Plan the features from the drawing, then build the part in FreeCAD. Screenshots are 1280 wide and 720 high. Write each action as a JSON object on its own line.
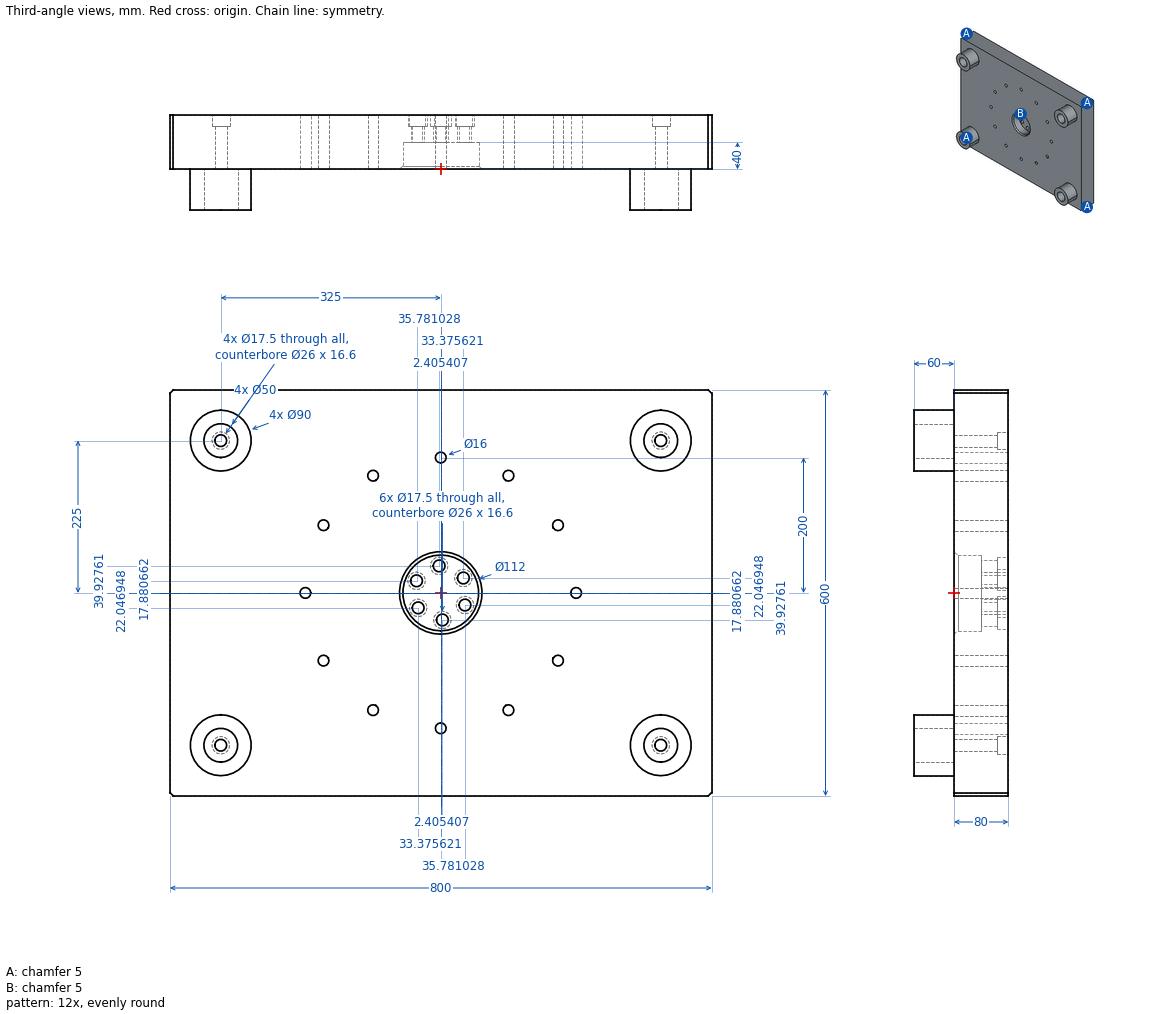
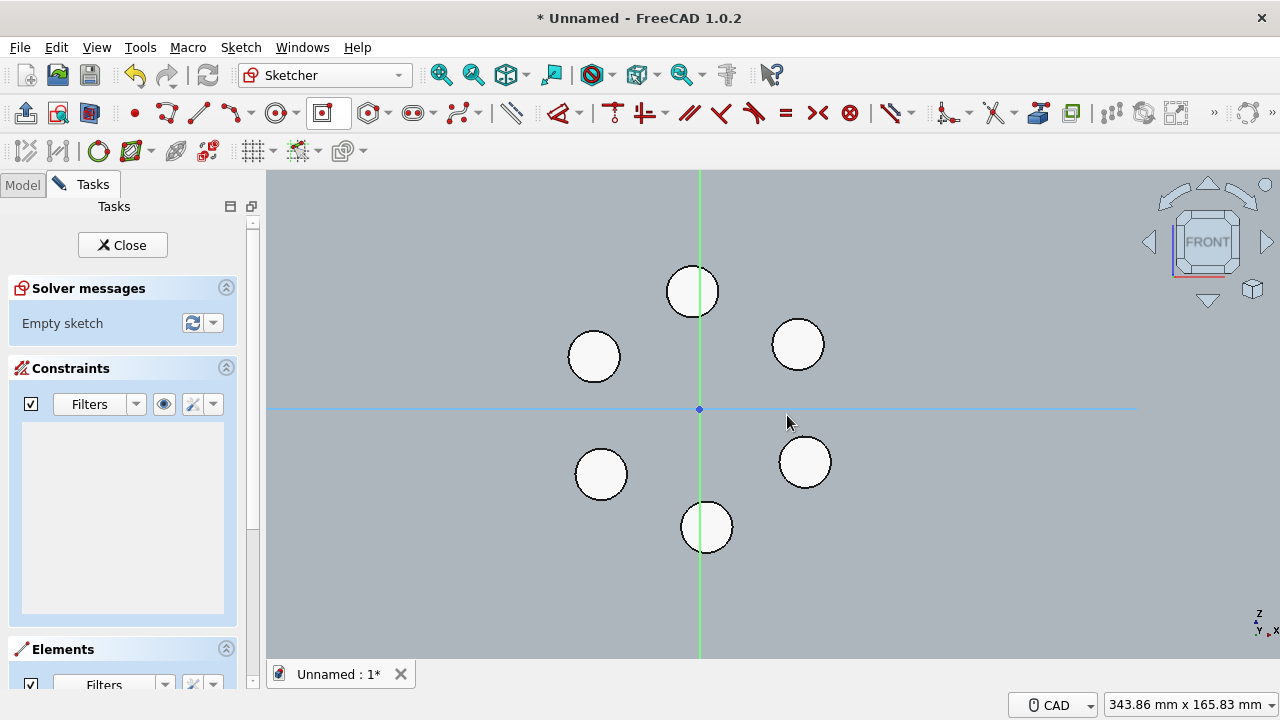
{"action": "left_click", "coordinate": [276, 114]}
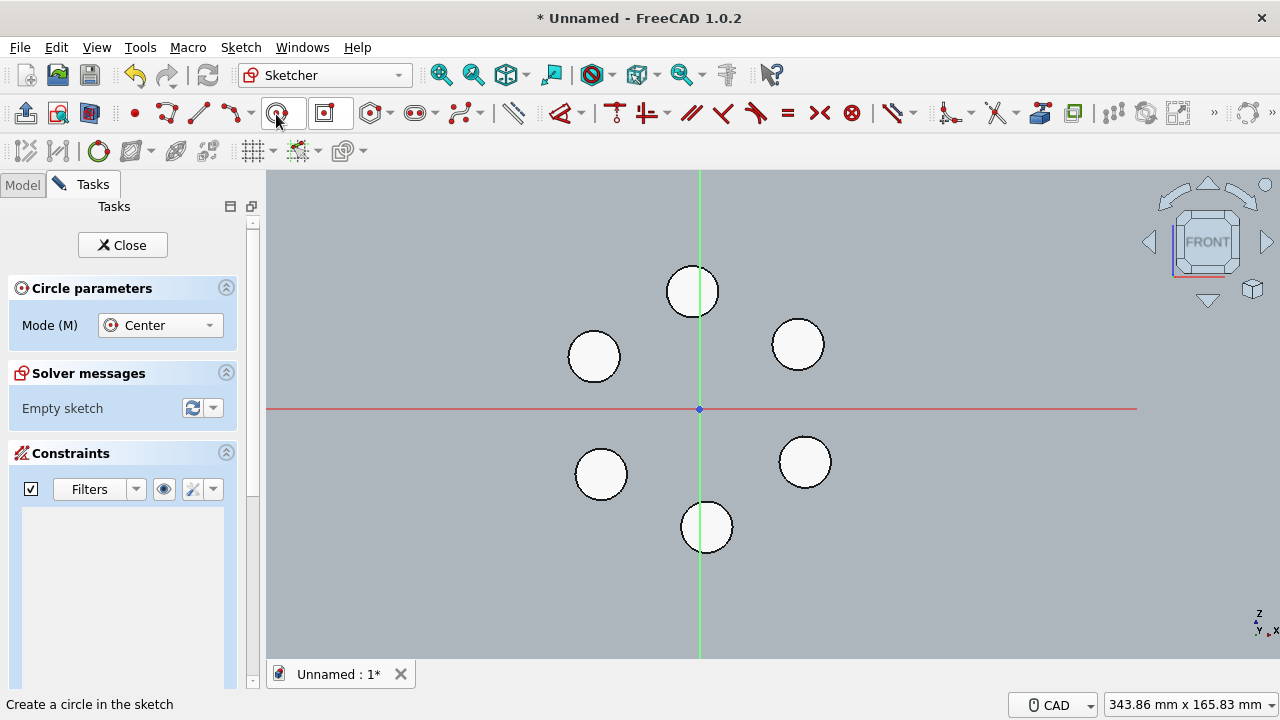
{"action": "left_click", "coordinate": [700, 409]}
{"action": "mouse_move", "coordinate": [816, 293]}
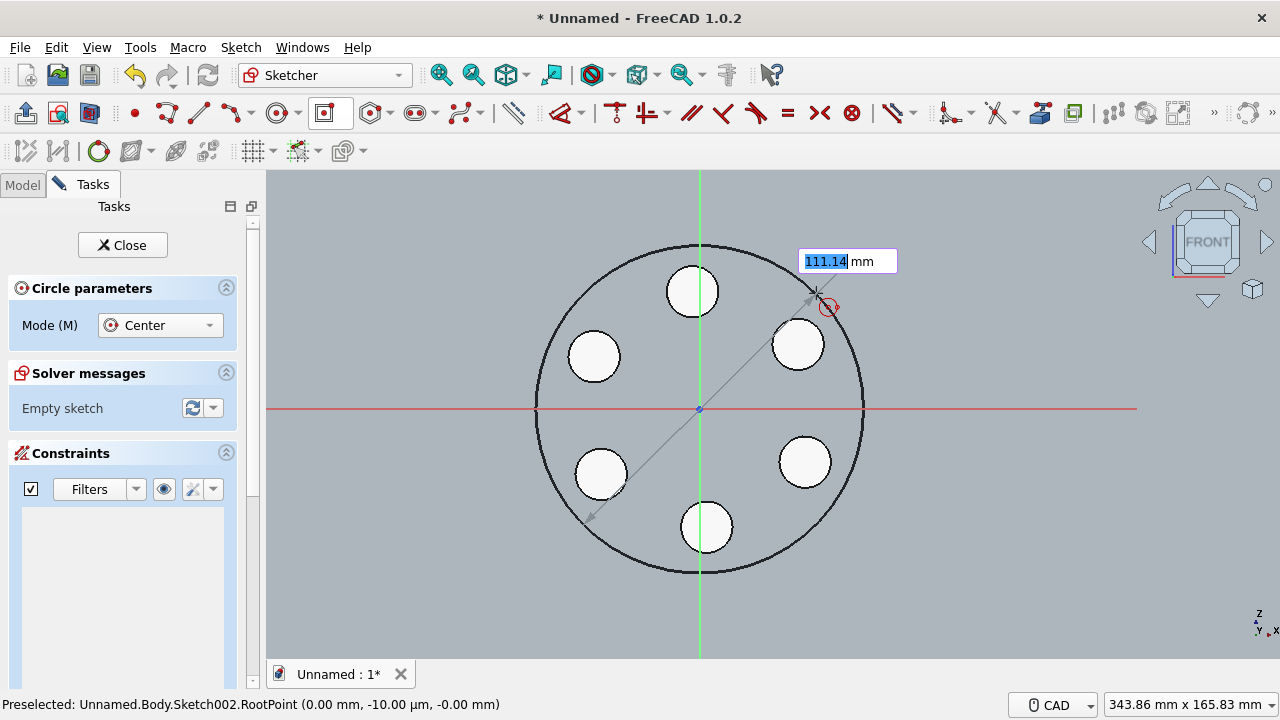
{"action": "type", "text": "112"}
{"action": "key", "text": "Return"}
{"action": "key", "text": "Escape"}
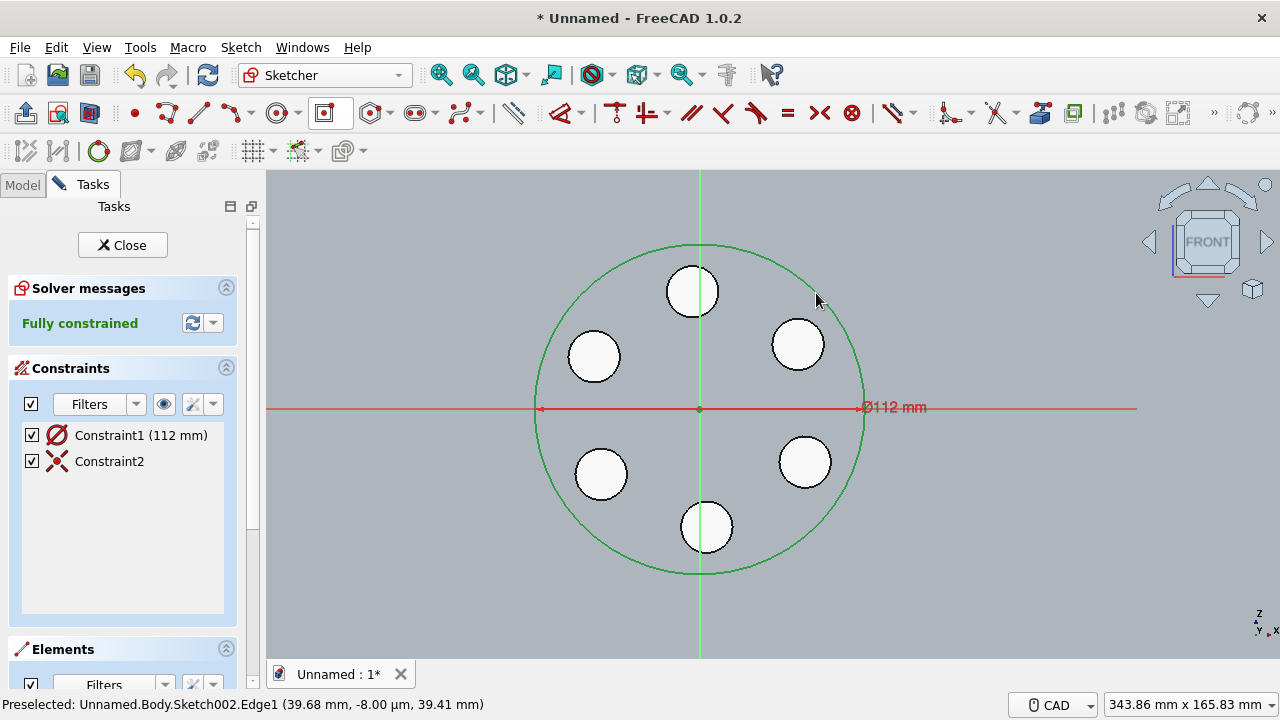
{"action": "left_click", "coordinate": [123, 245]}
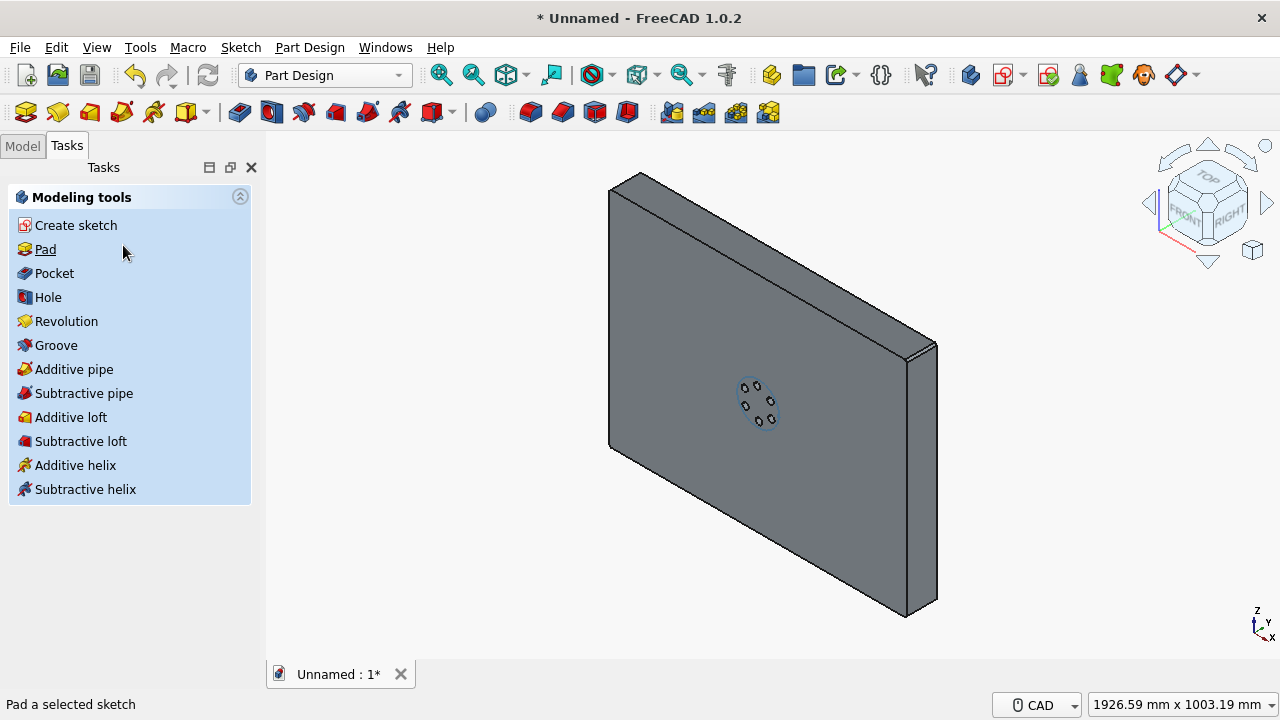
{"action": "left_click", "coordinate": [240, 112]}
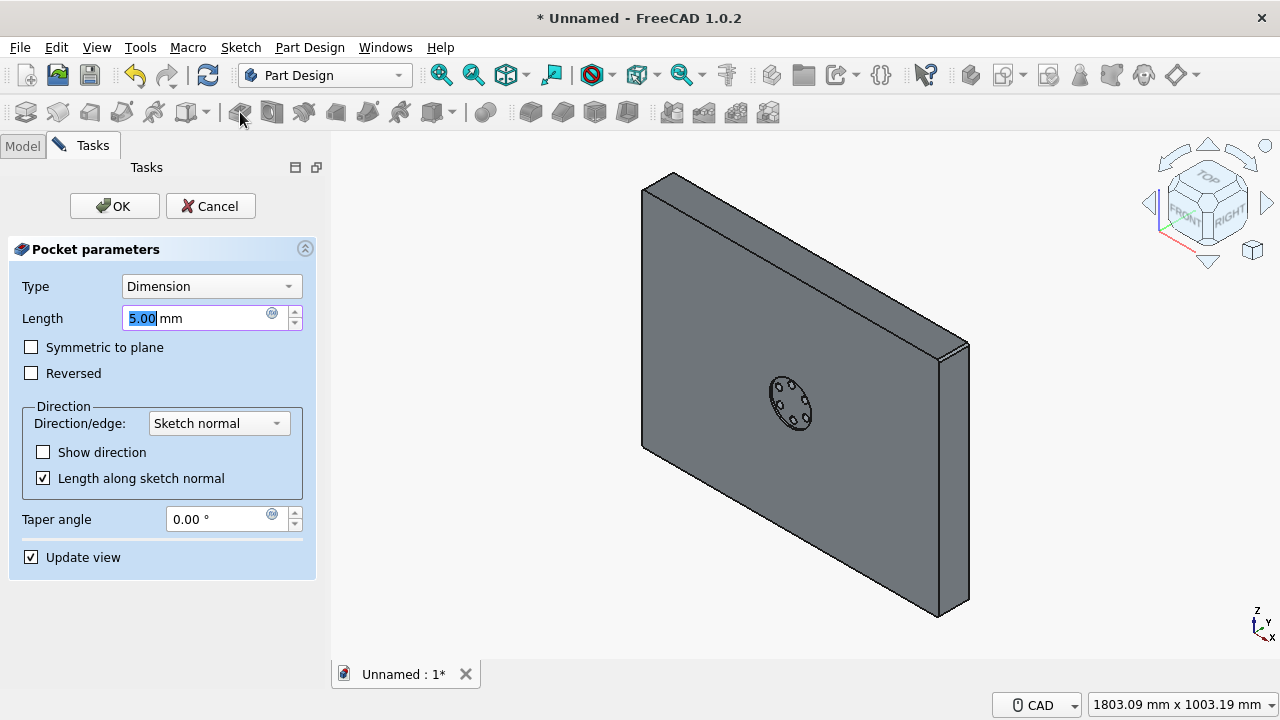
{"action": "type", "text": "40"}
{"action": "key", "text": "Tab"}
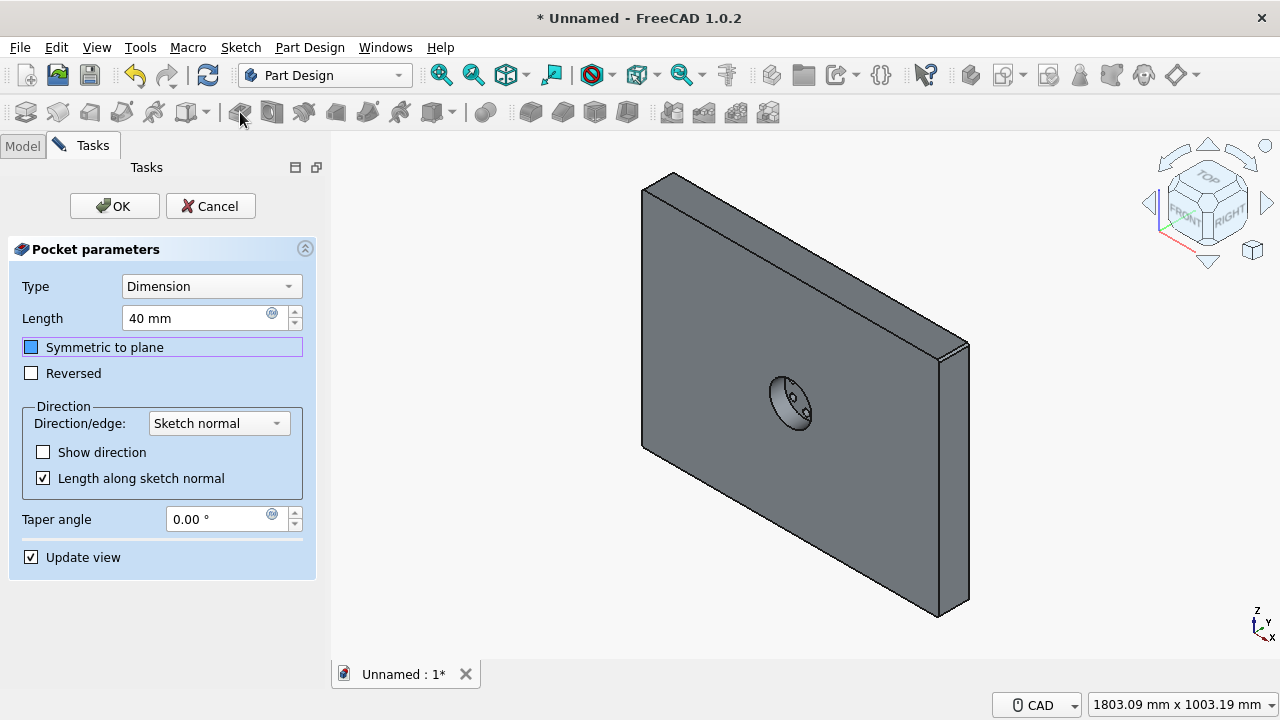
{"action": "left_click", "coordinate": [115, 206]}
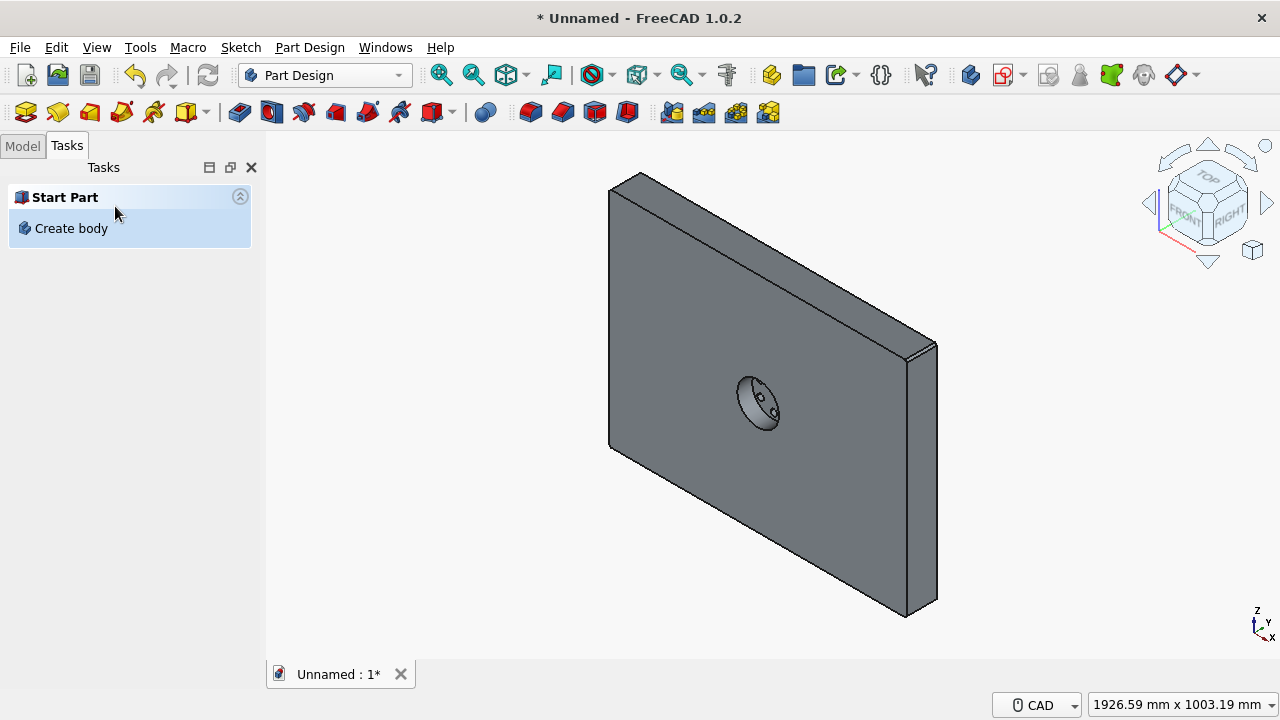
{"action": "left_click", "coordinate": [737, 391]}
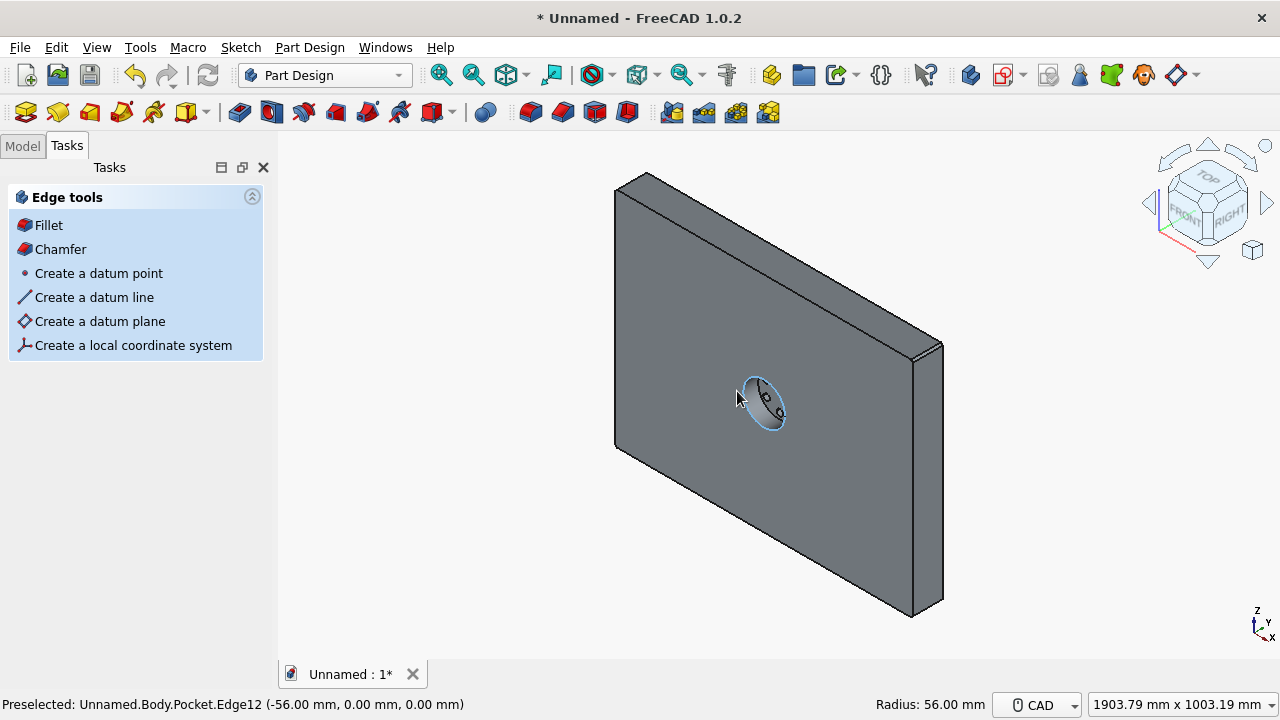
{"action": "left_click", "coordinate": [564, 112]}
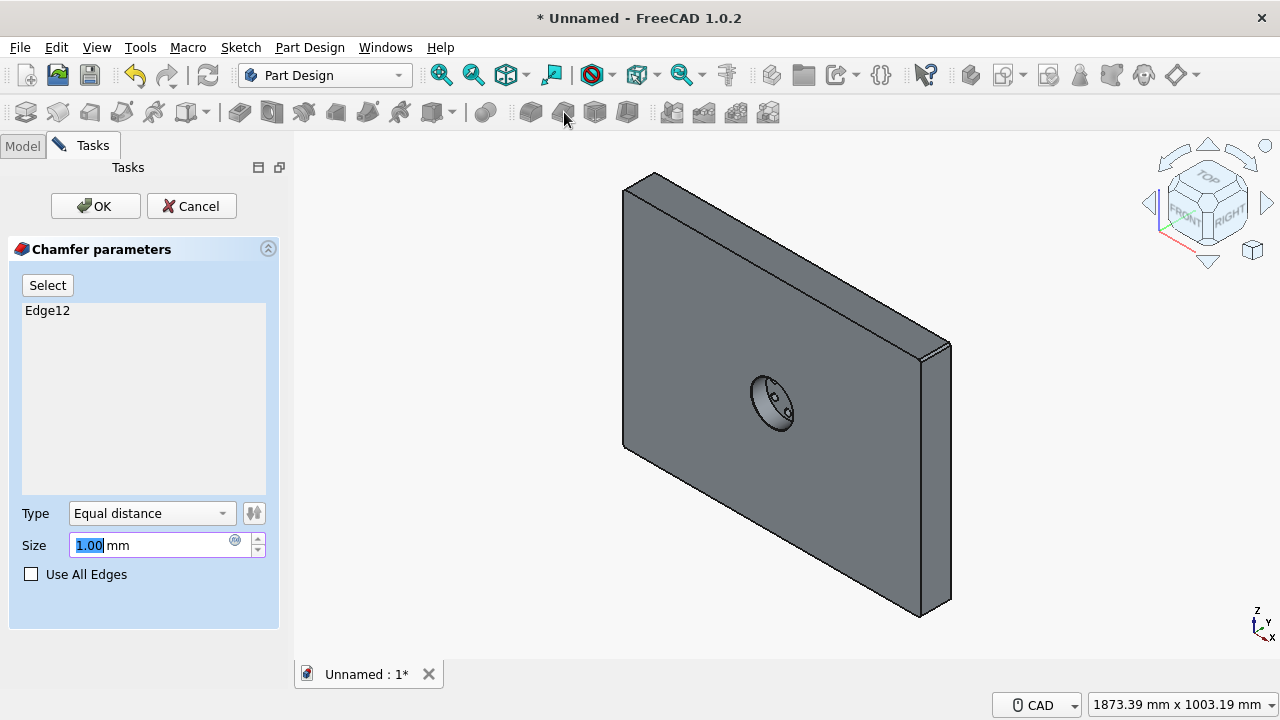
{"action": "type", "text": "5"}
{"action": "key", "text": "Tab"}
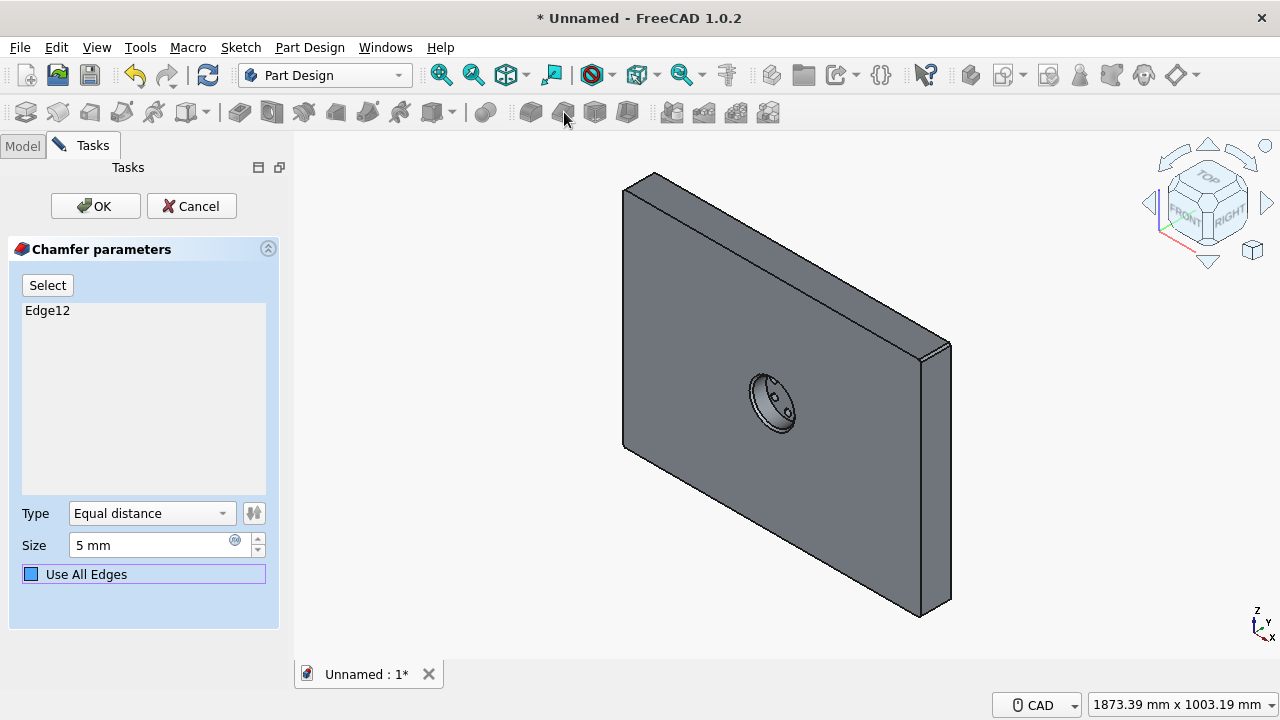
{"action": "left_click", "coordinate": [96, 206]}